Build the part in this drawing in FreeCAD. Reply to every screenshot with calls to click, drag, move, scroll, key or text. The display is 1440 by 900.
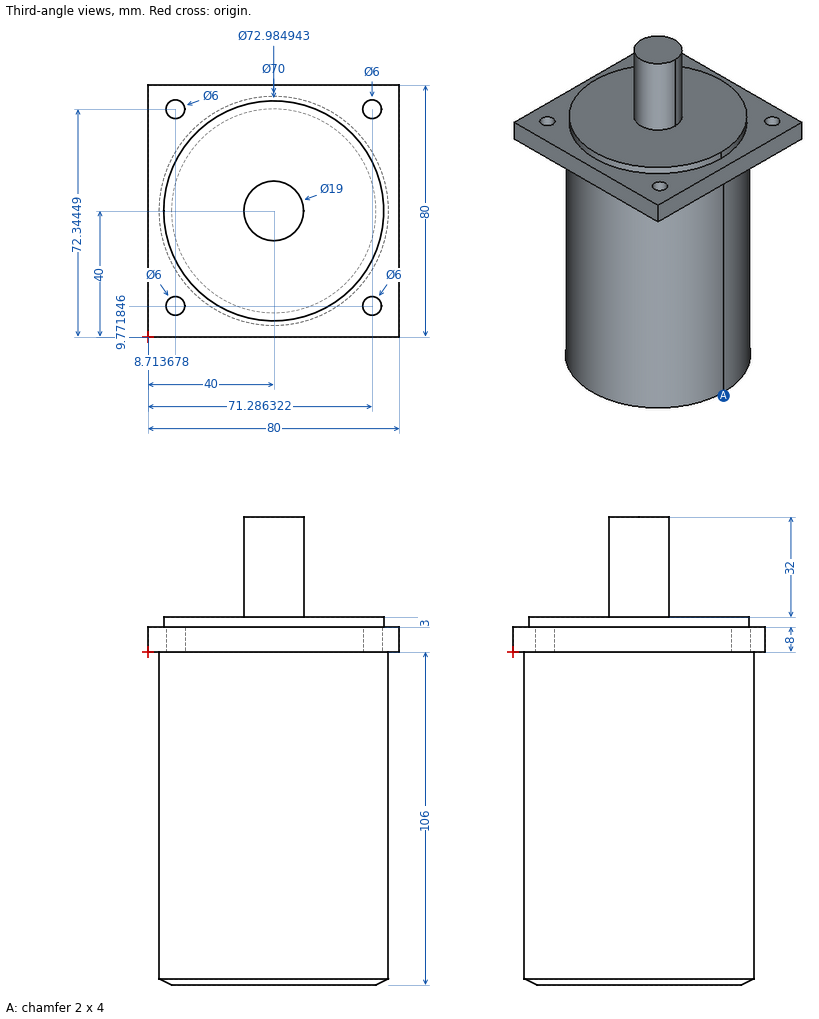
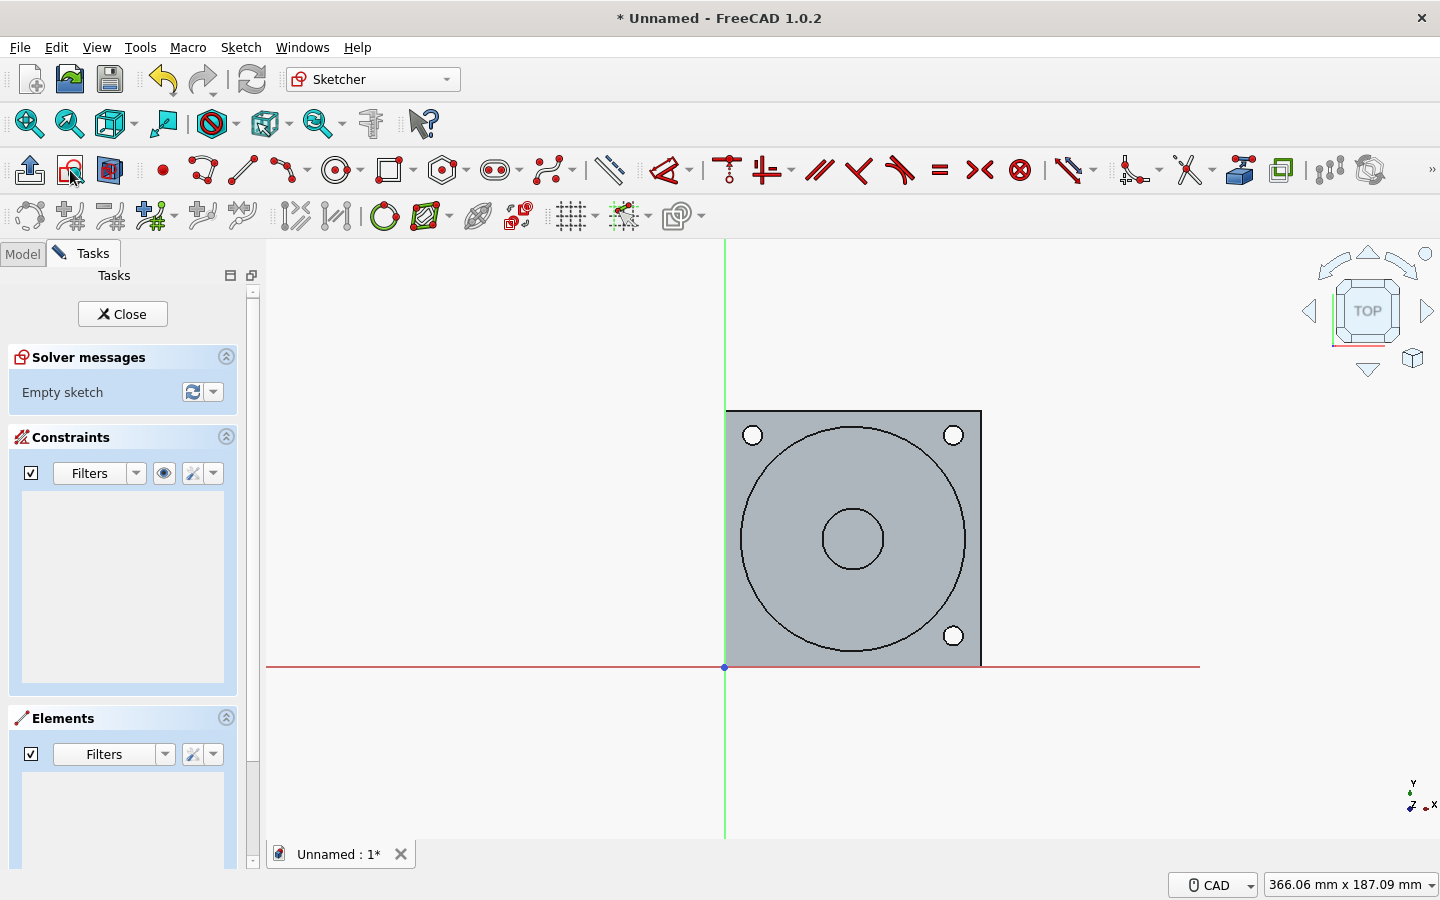
click(110, 170)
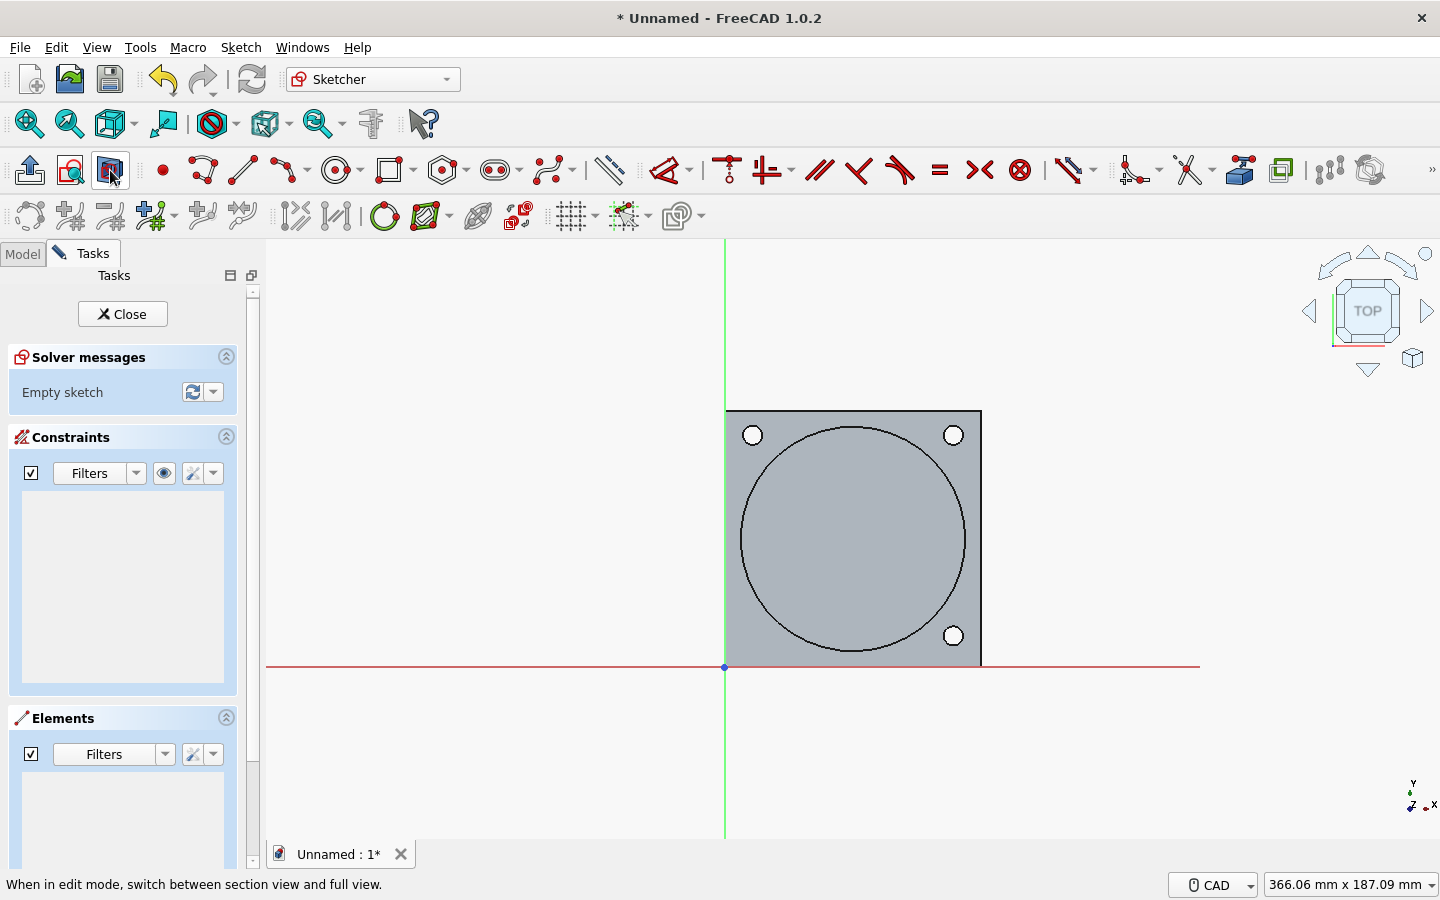
scroll(738, 660, up, 11)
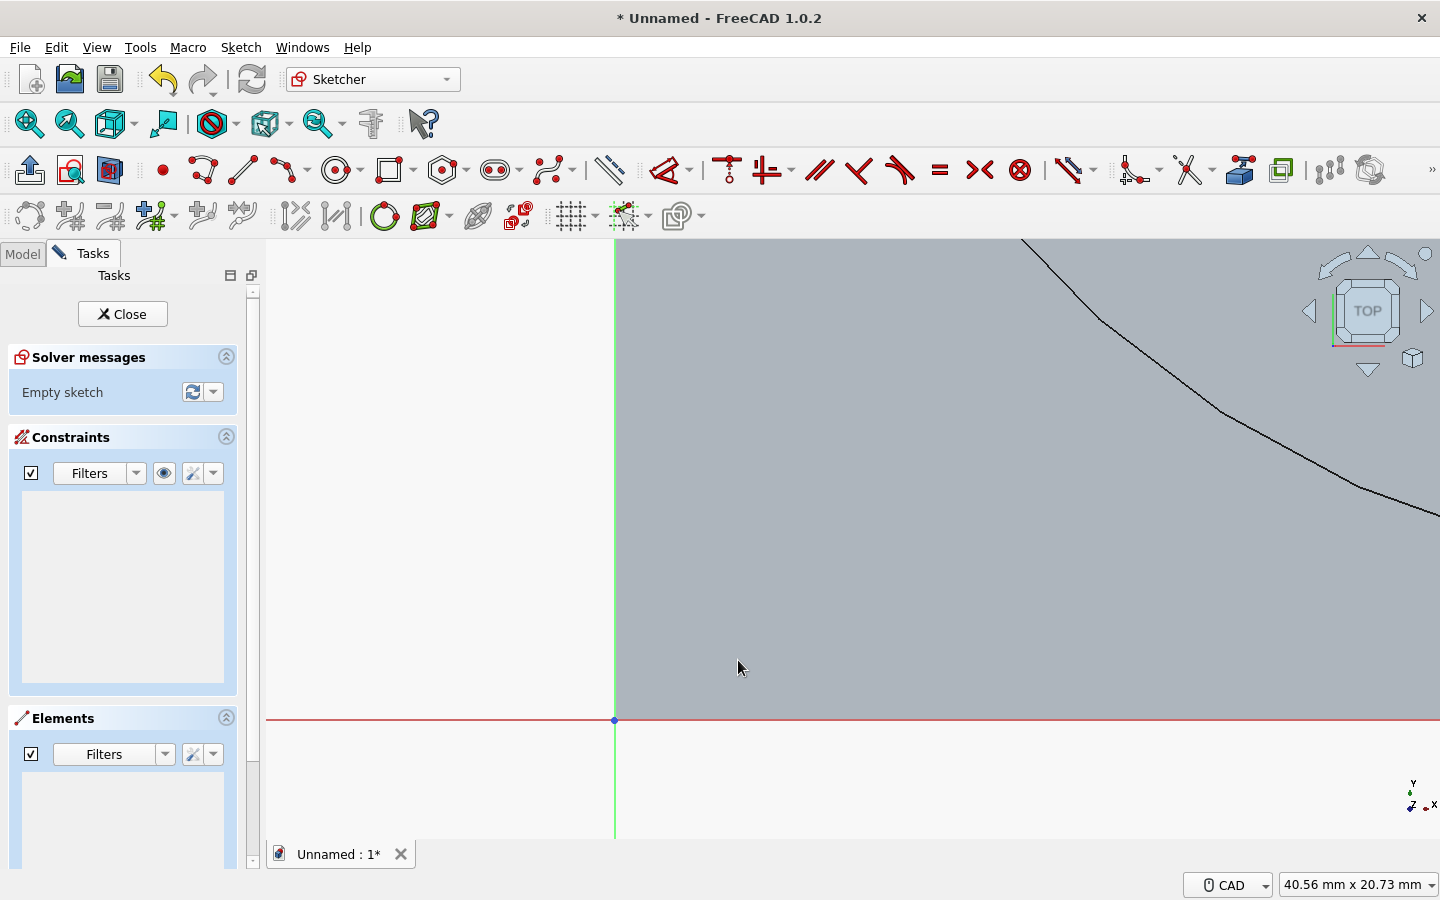
click(336, 170)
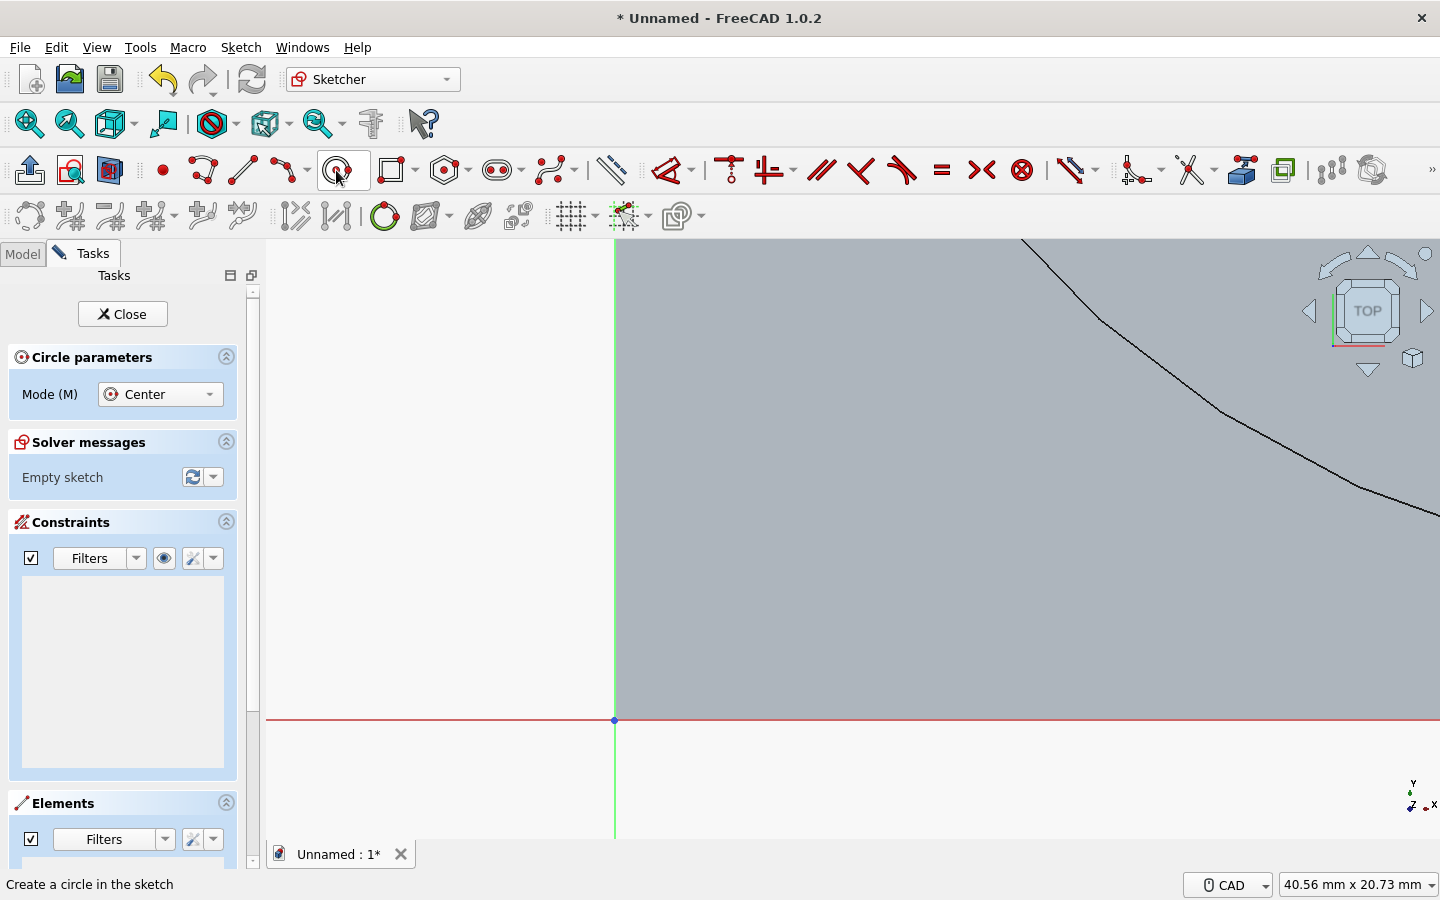
click(867, 437)
move(928, 376)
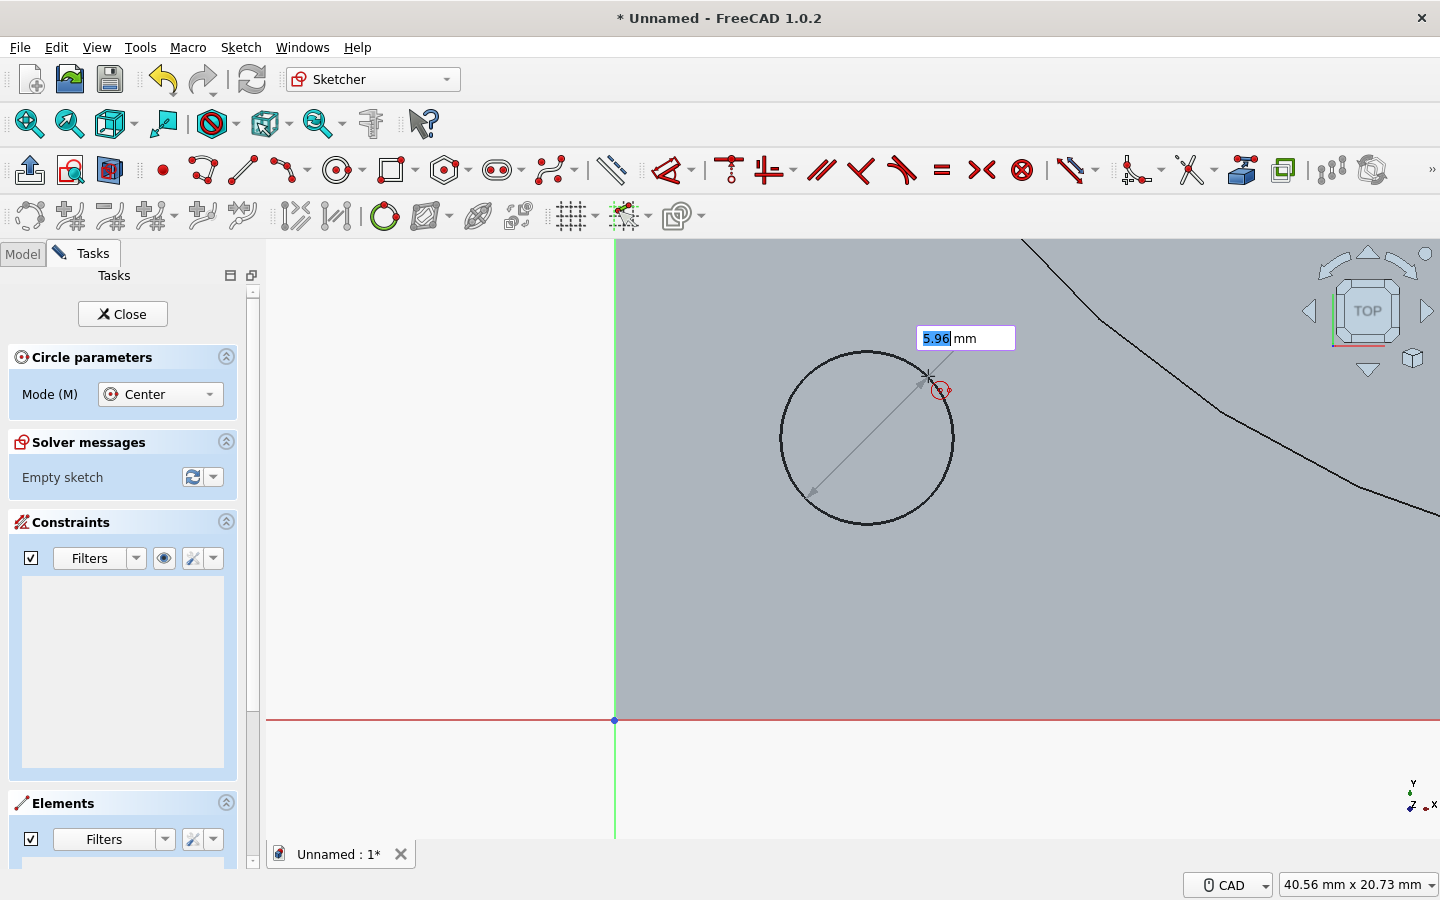
text(6)
key(Return)
key(Escape)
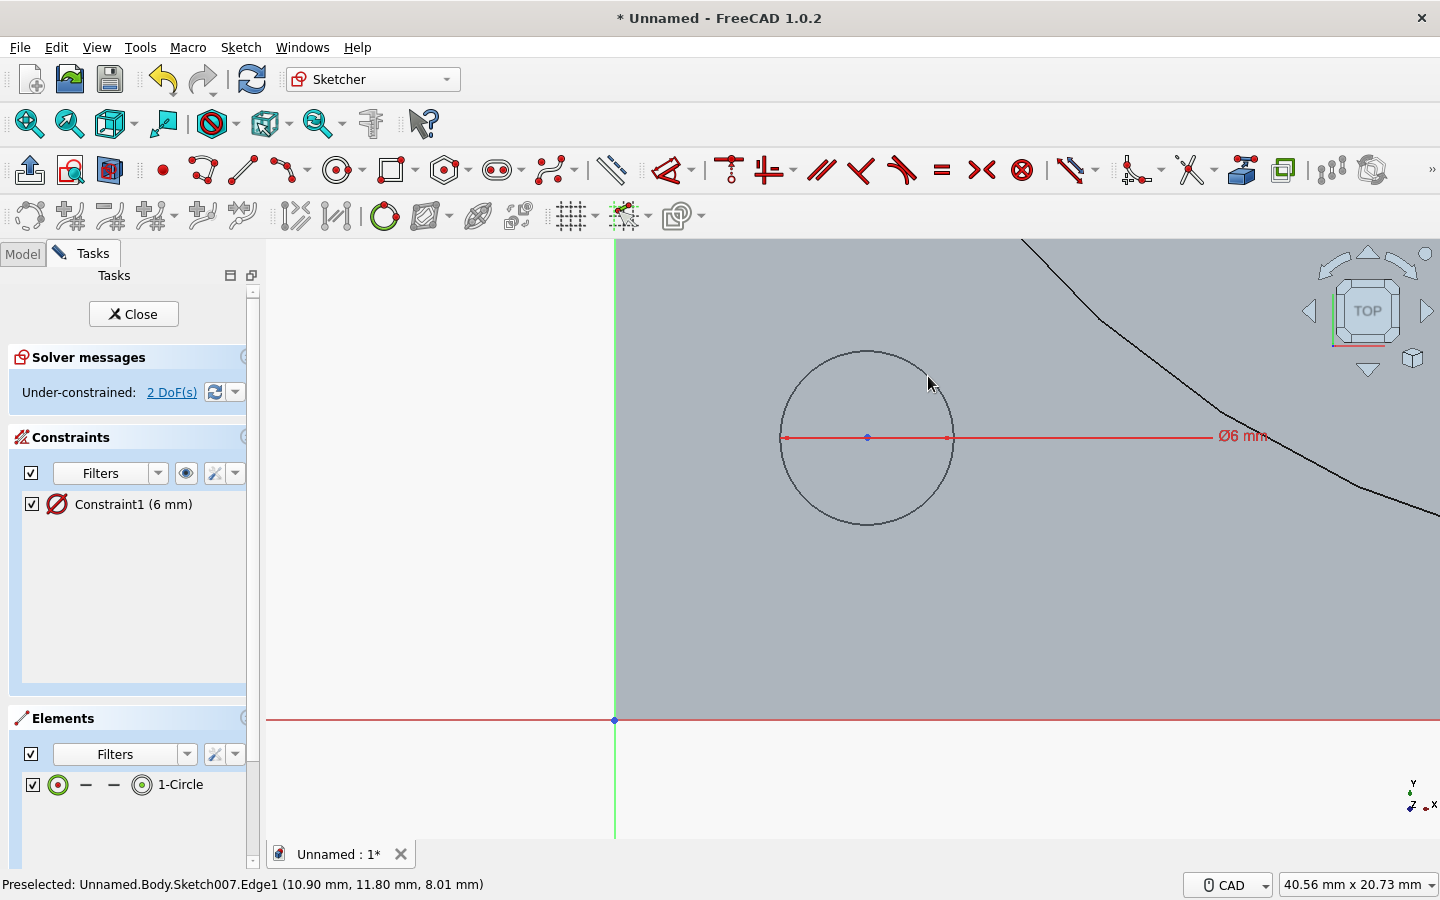
click(666, 170)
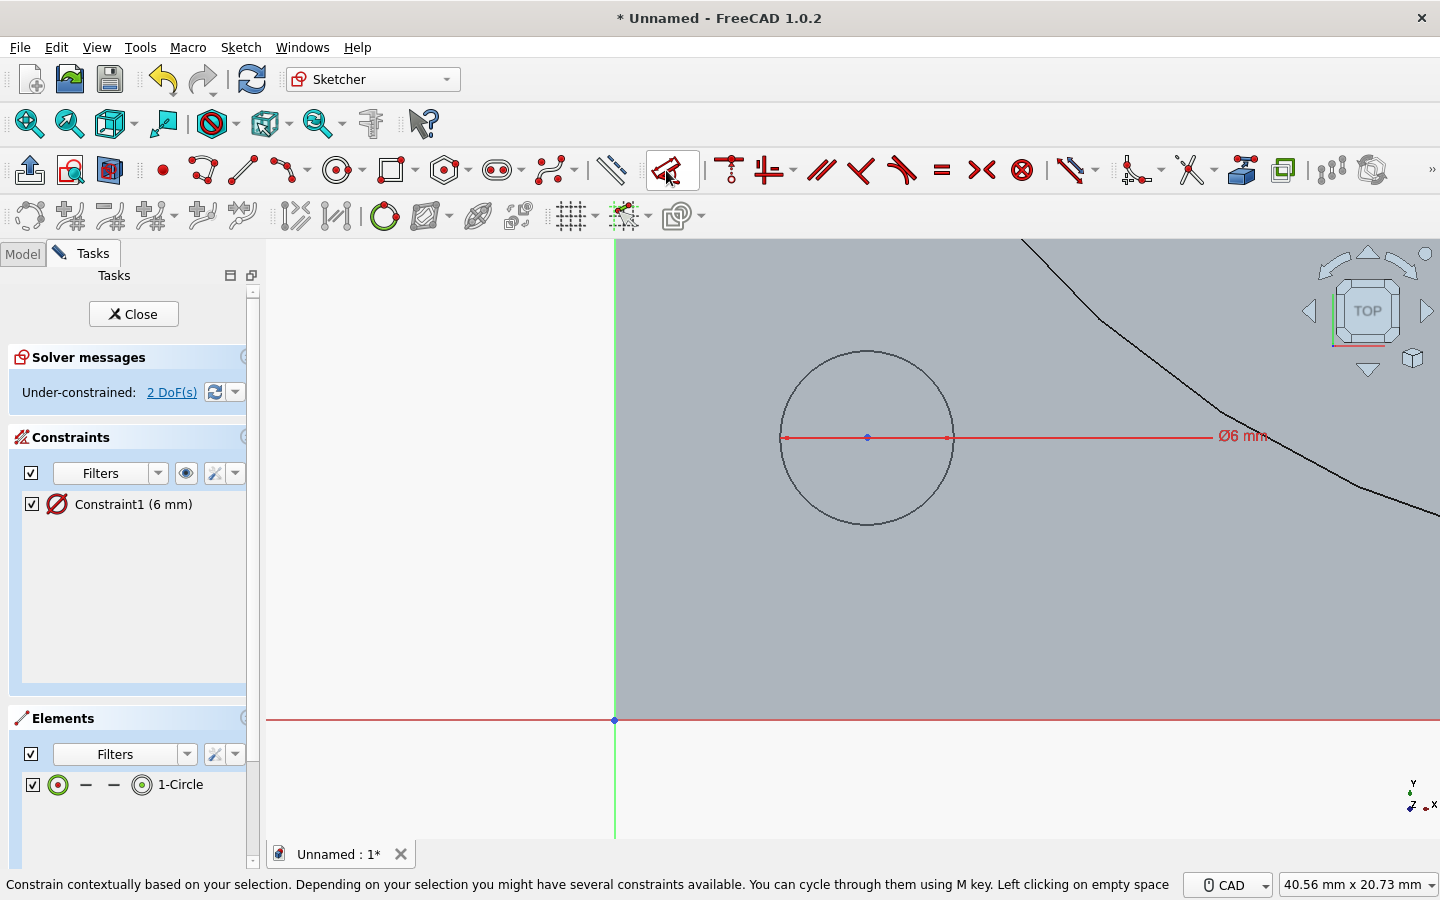
click(867, 438)
click(741, 754)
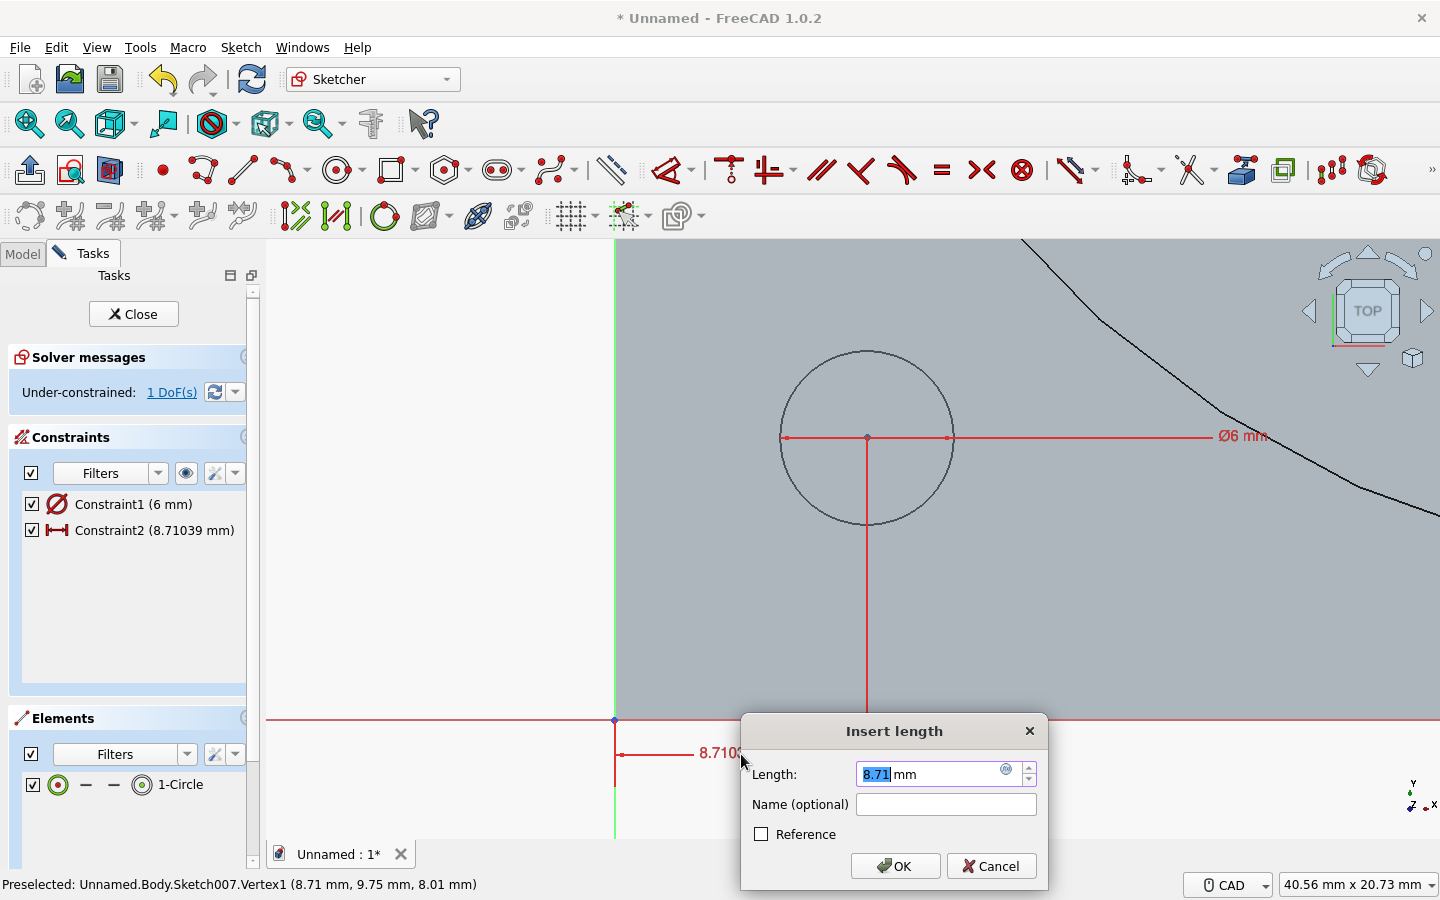
text(8.713678)
key(Return)